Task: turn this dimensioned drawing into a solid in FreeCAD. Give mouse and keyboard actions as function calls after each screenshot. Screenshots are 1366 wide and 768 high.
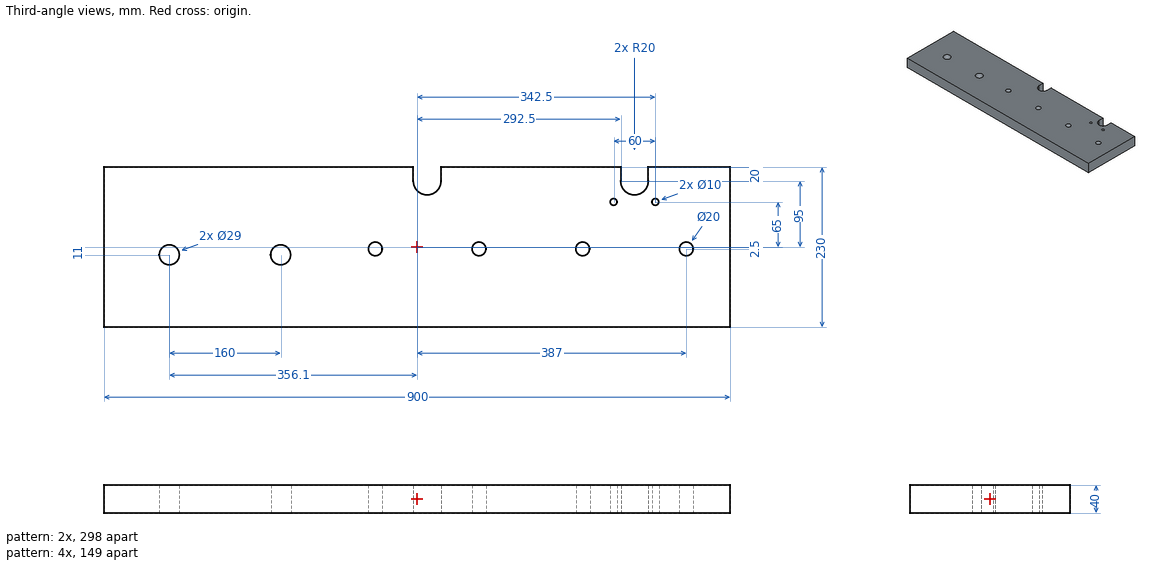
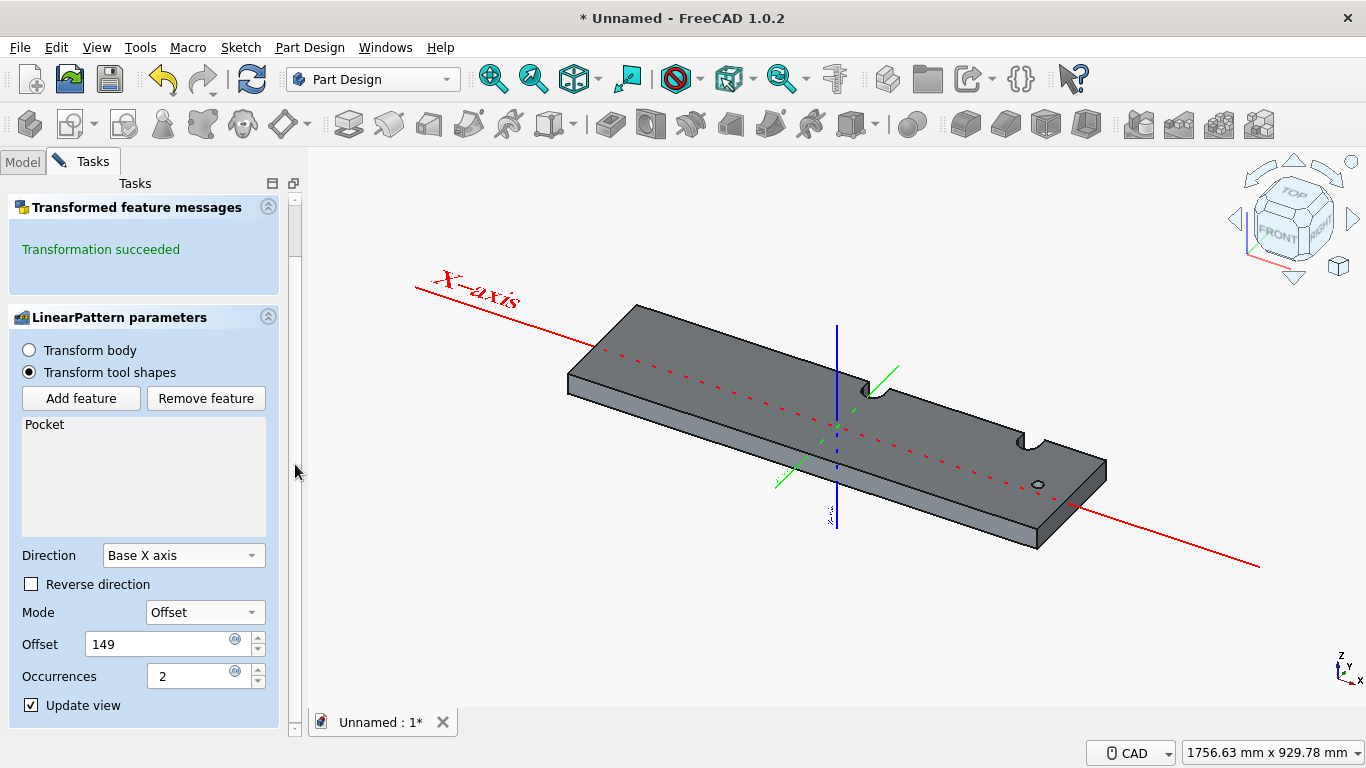
triple_click(198, 676)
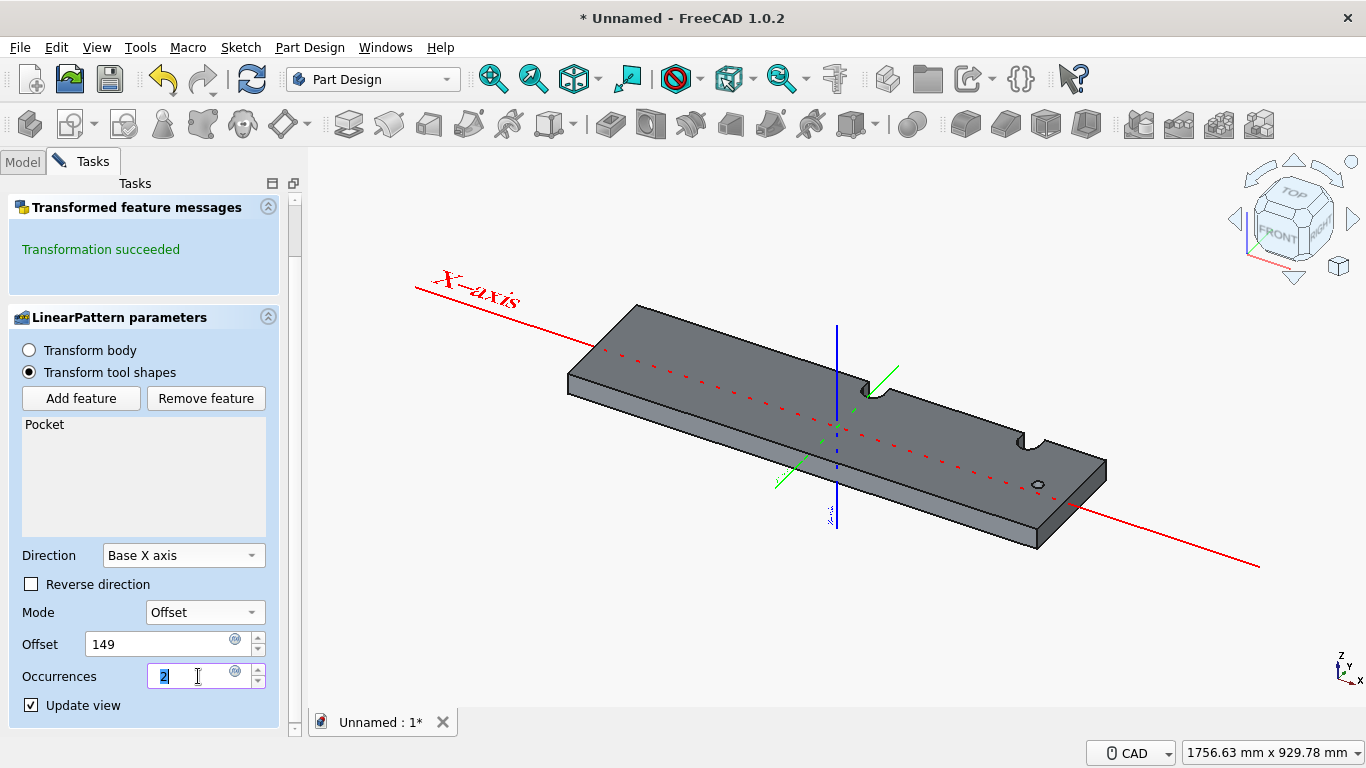
text(4)
key(Tab)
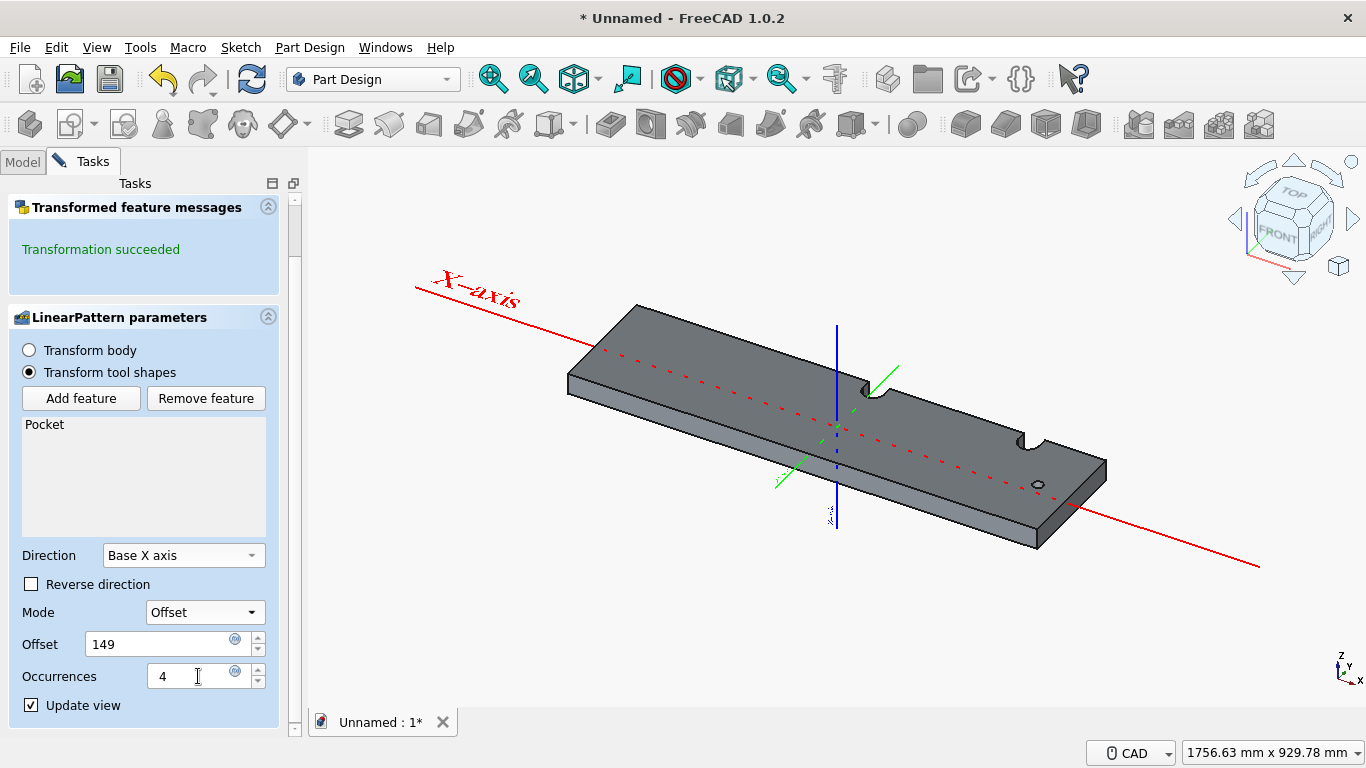
click(30, 584)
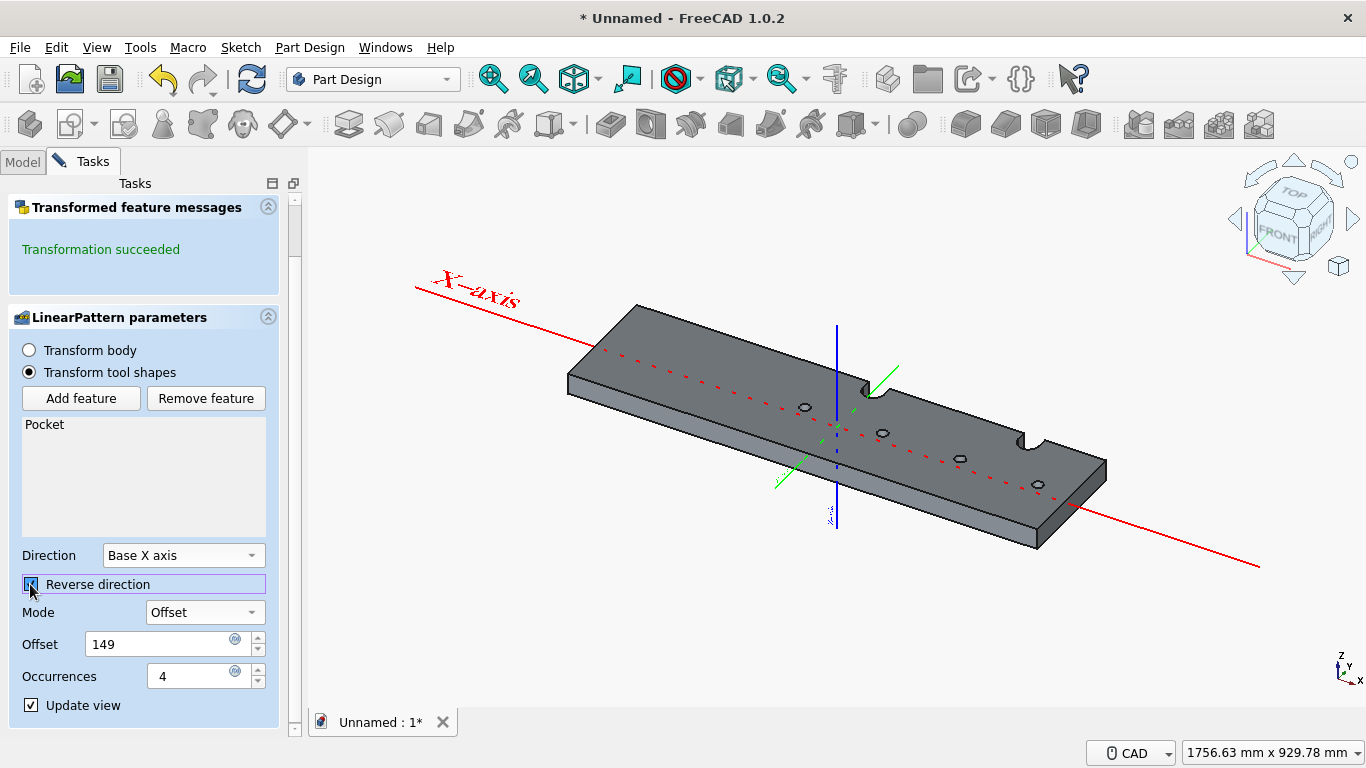
scroll(295, 464, up, 2)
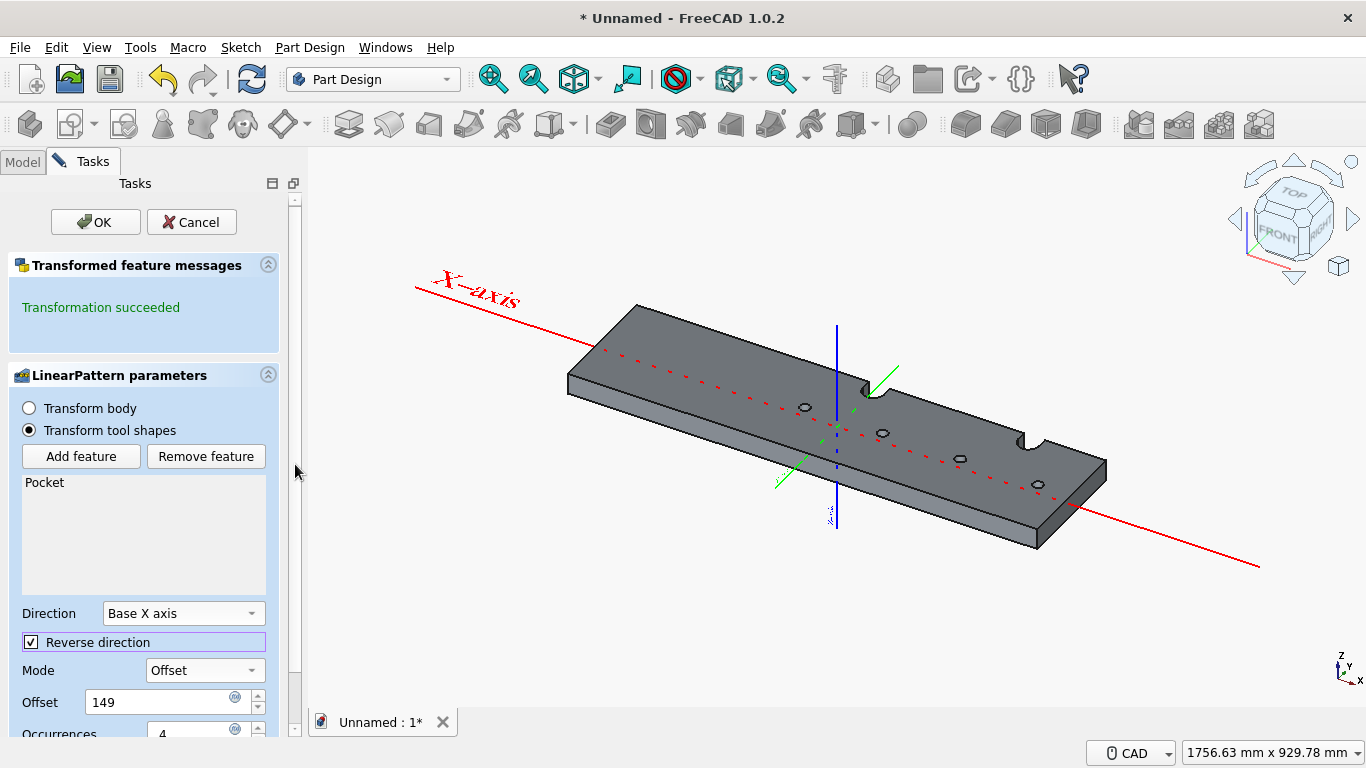
click(96, 222)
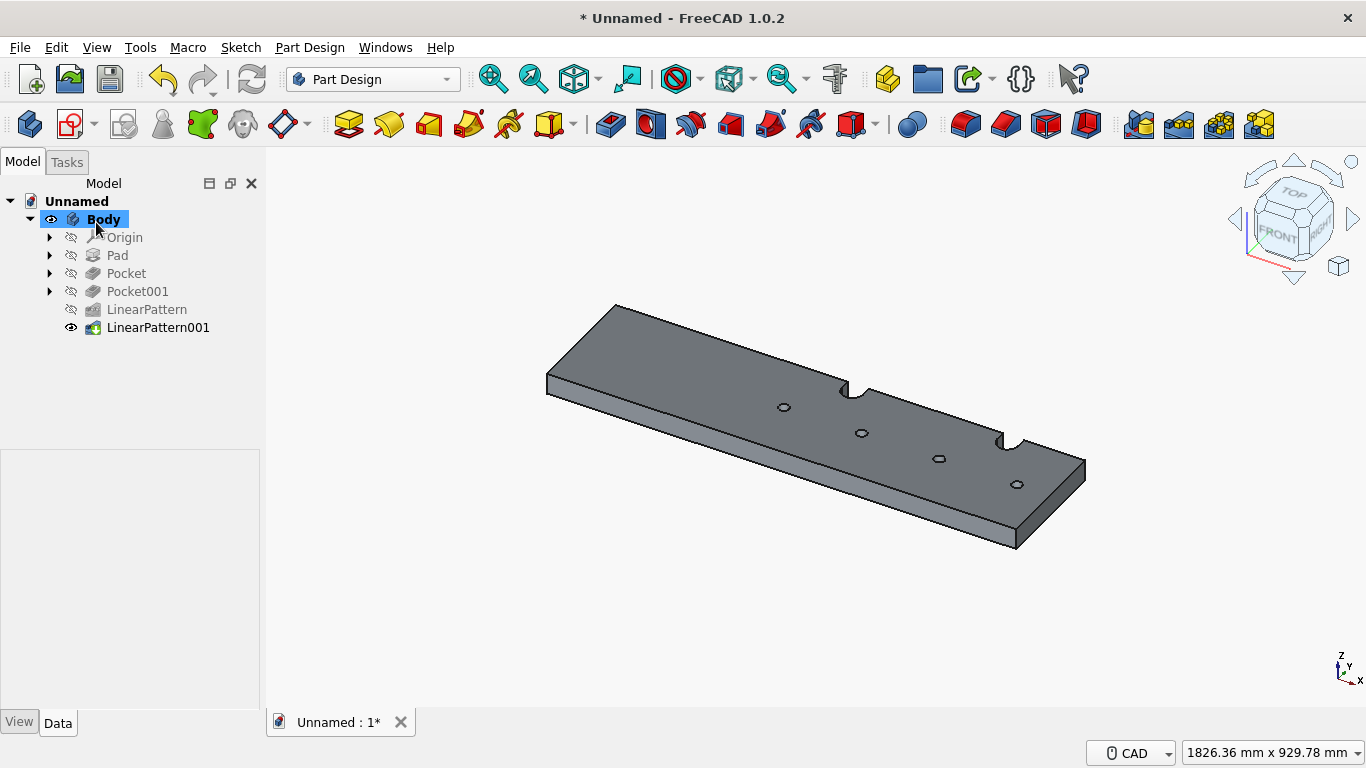
key(5)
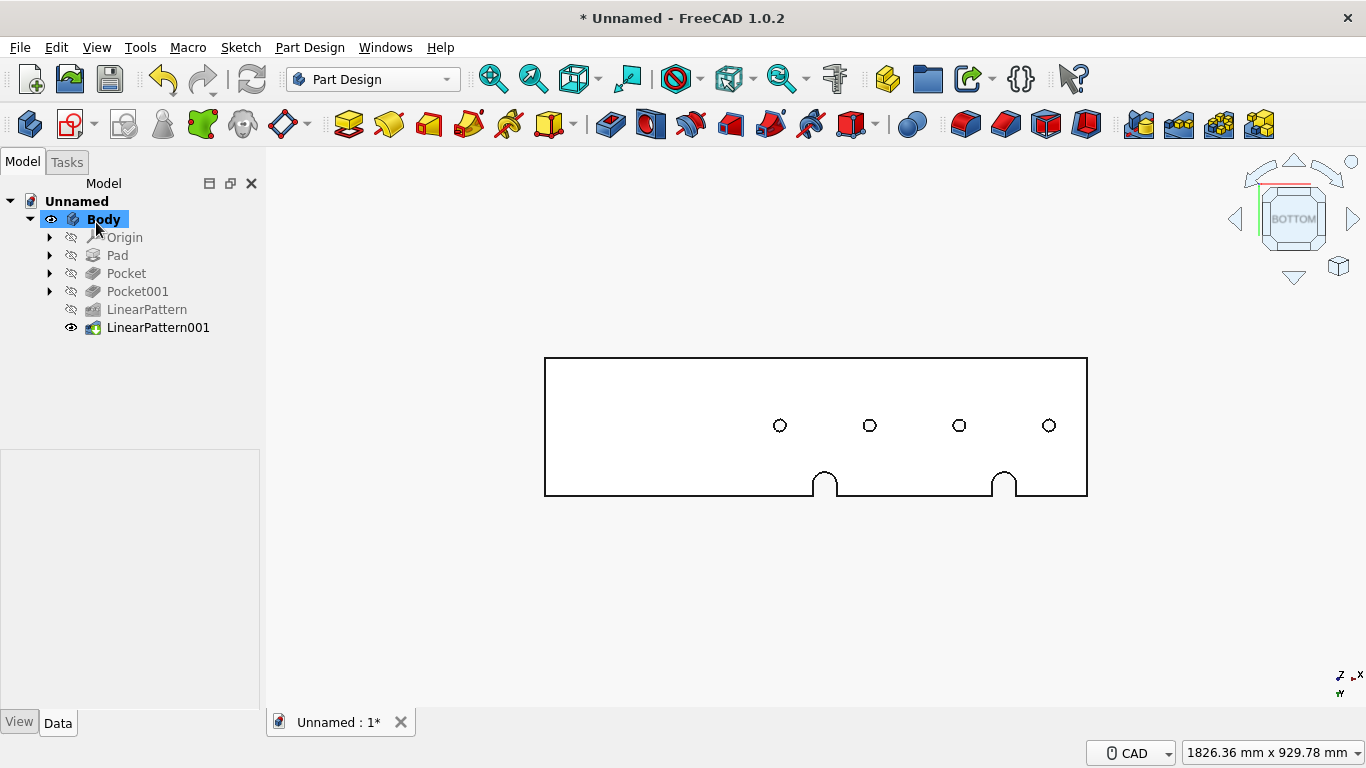
click(661, 426)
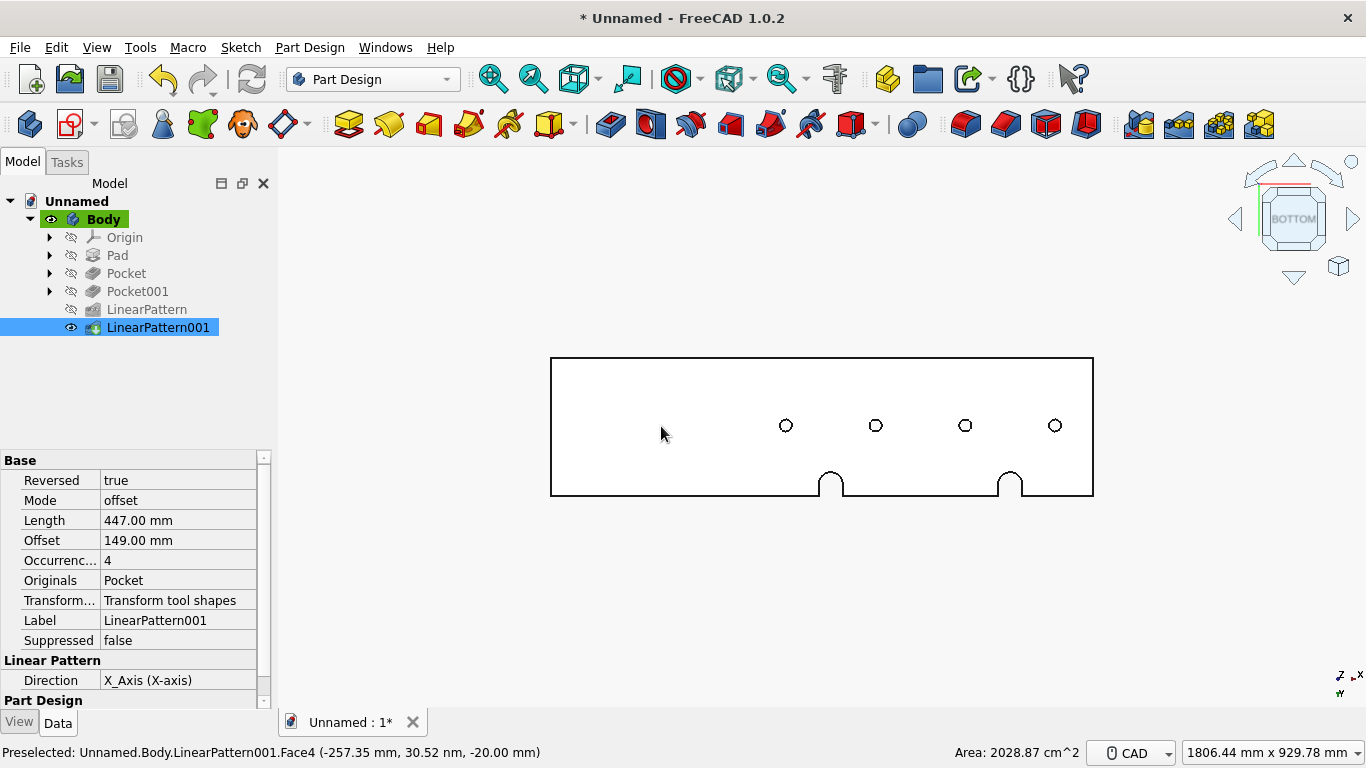
click(70, 124)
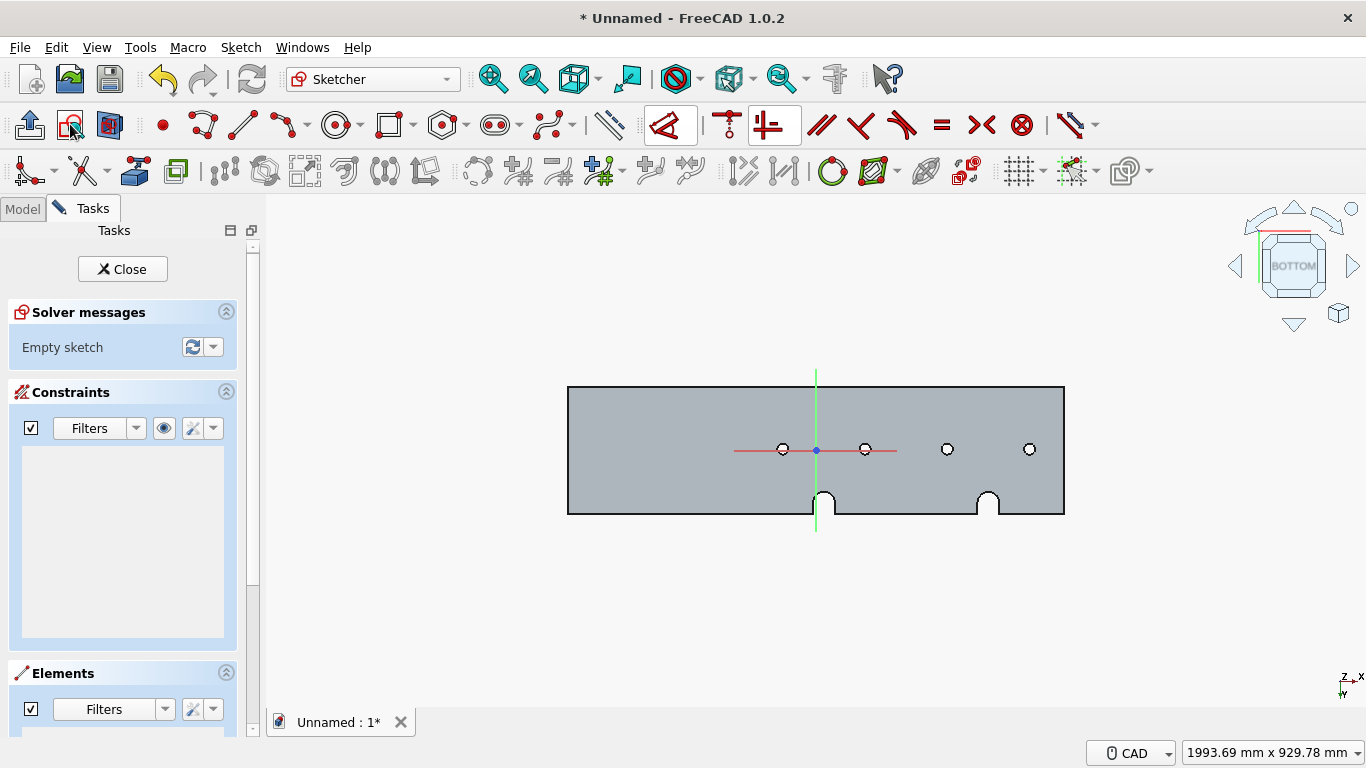
scroll(1004, 489, up, 14)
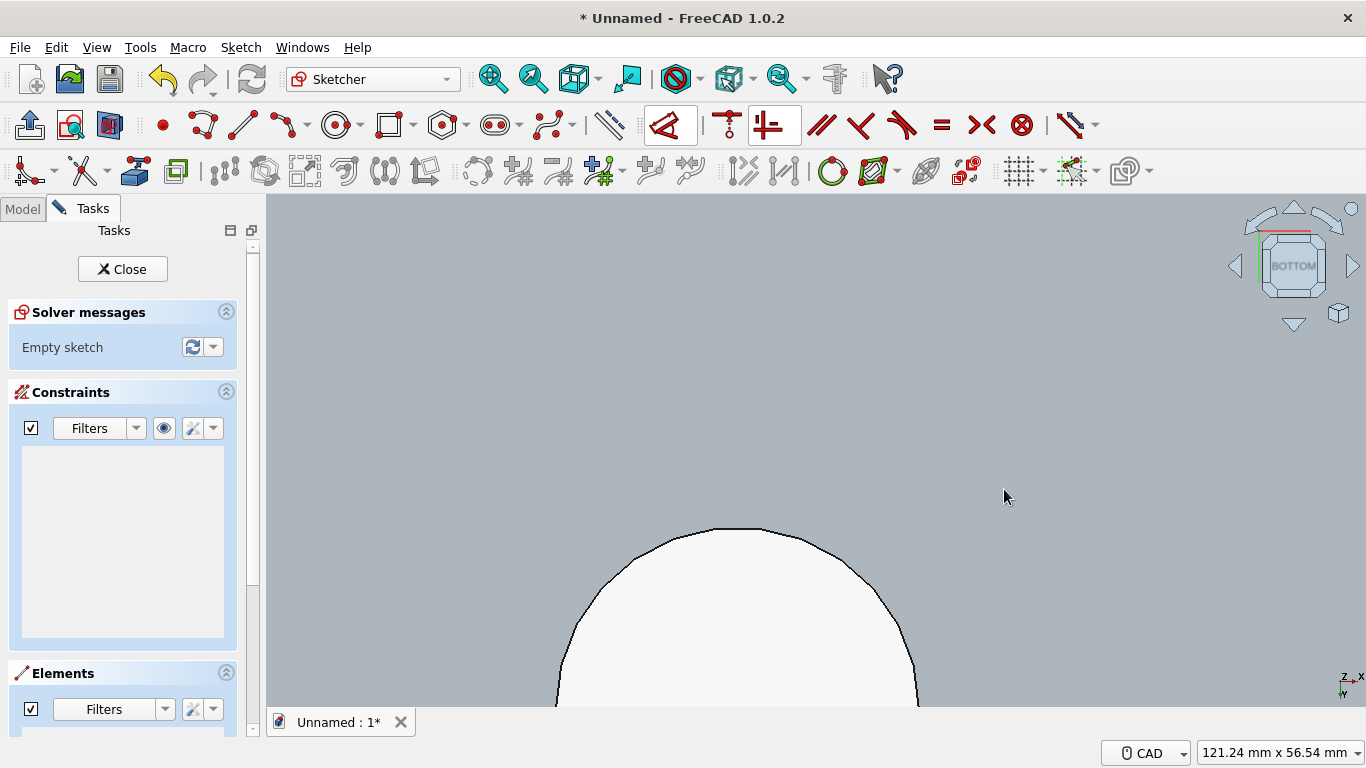
key(g)
key(c)